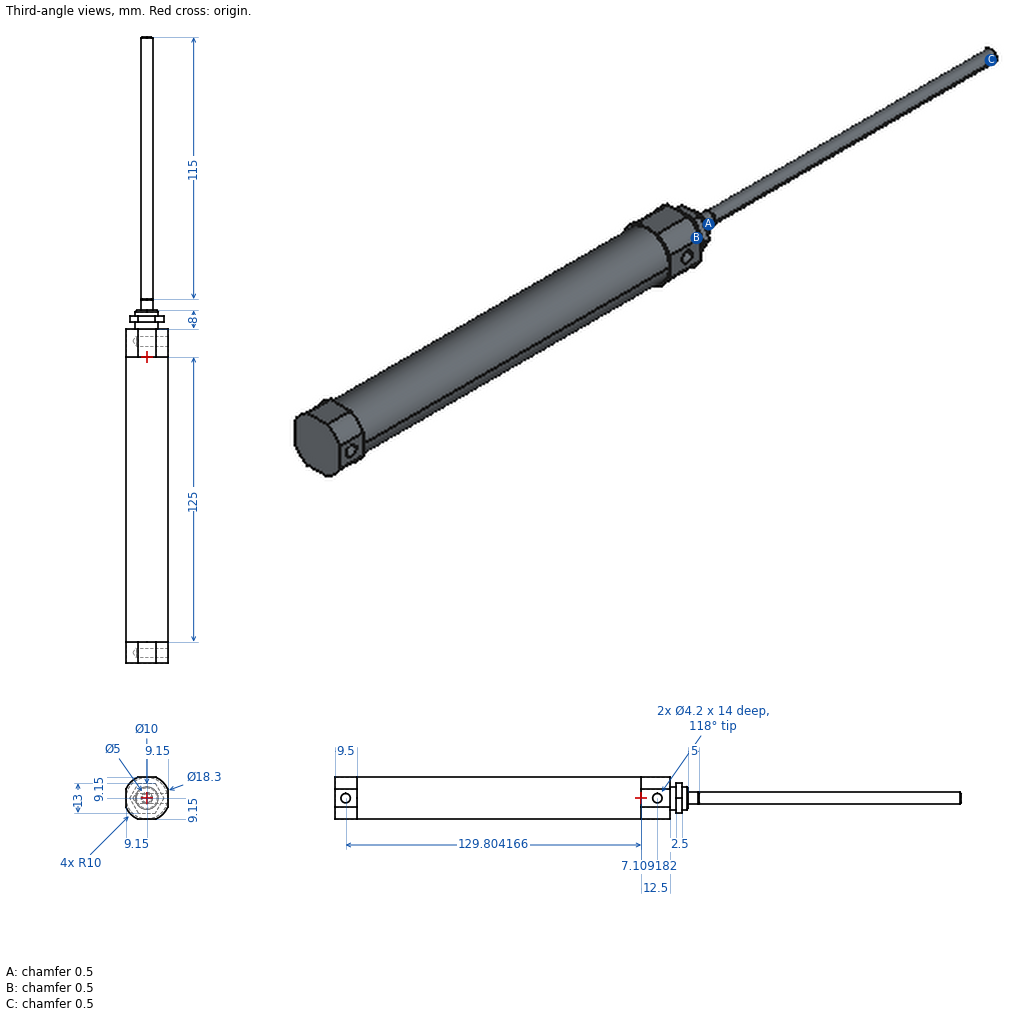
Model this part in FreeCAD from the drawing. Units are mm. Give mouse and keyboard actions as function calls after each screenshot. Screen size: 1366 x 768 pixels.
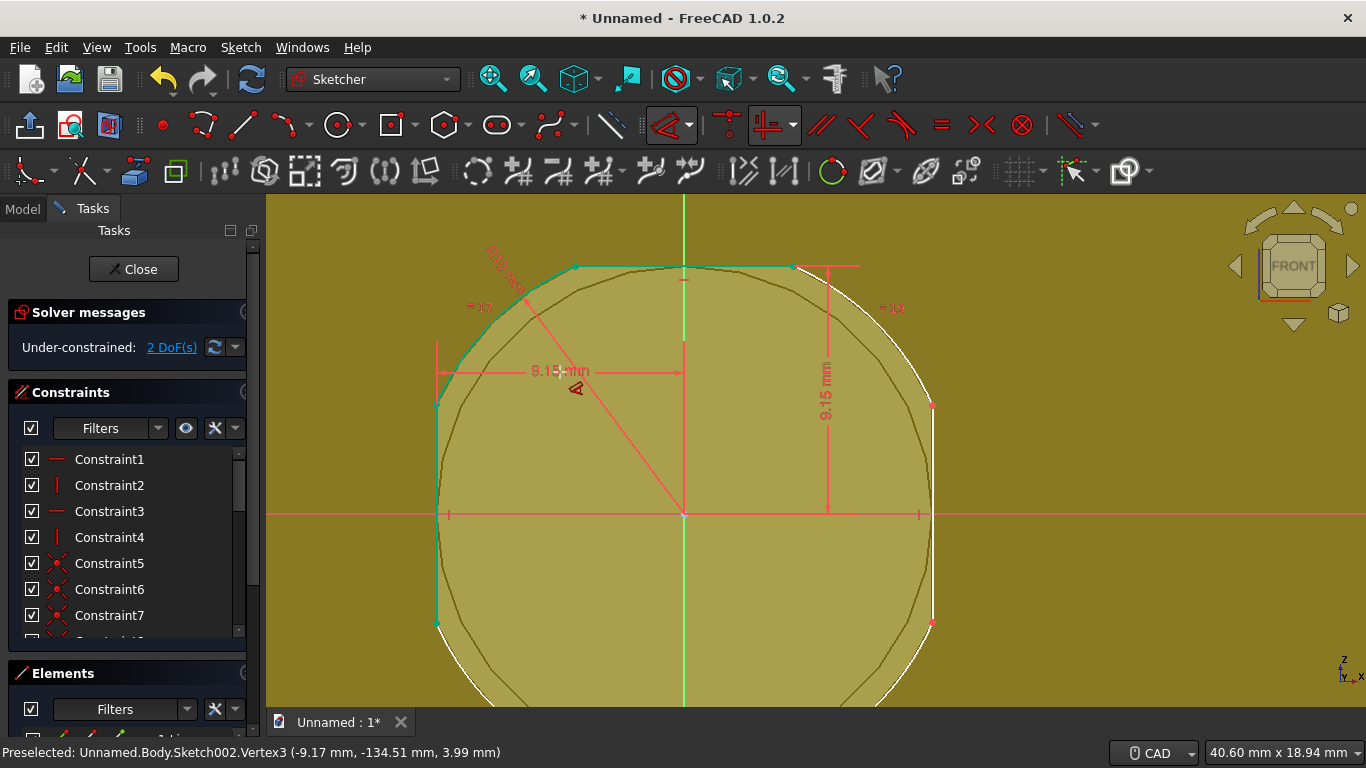
scroll(876, 321, down, 2)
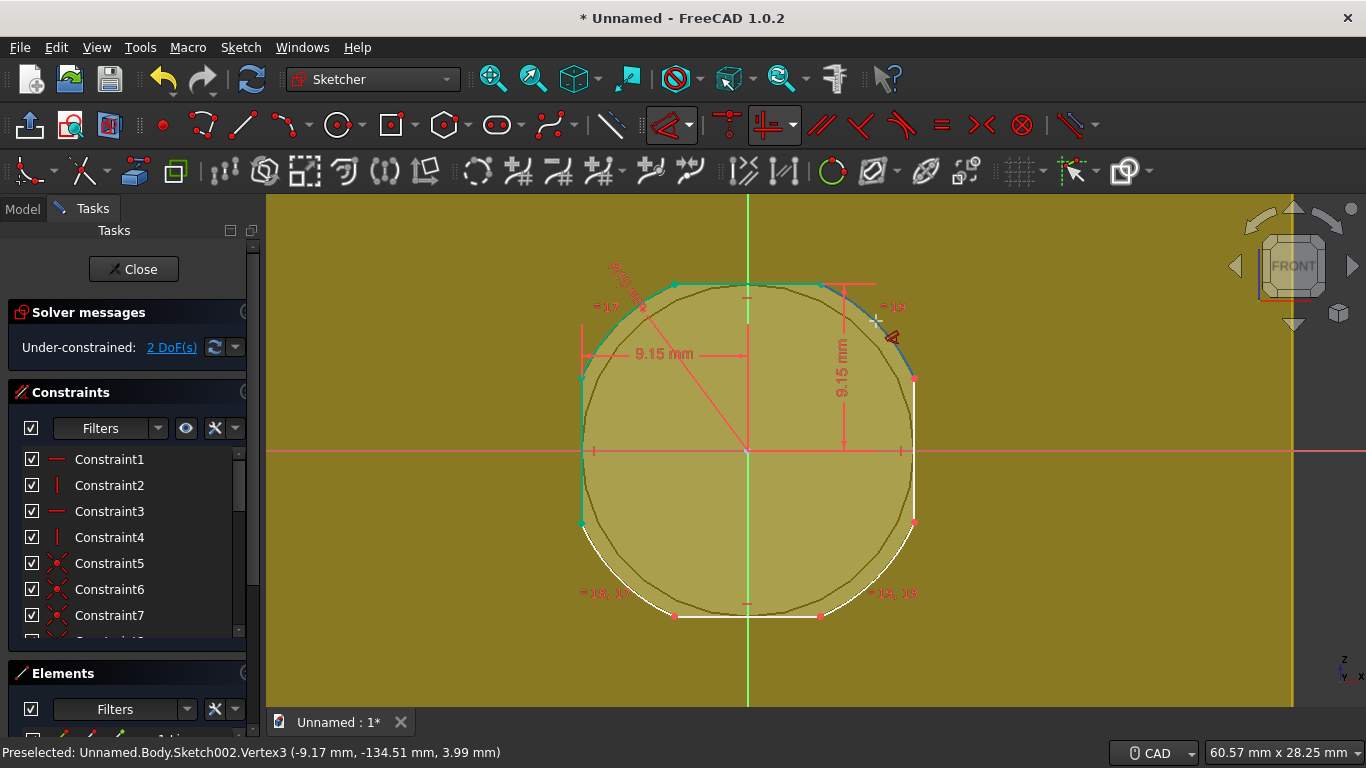
click(675, 617)
click(641, 534)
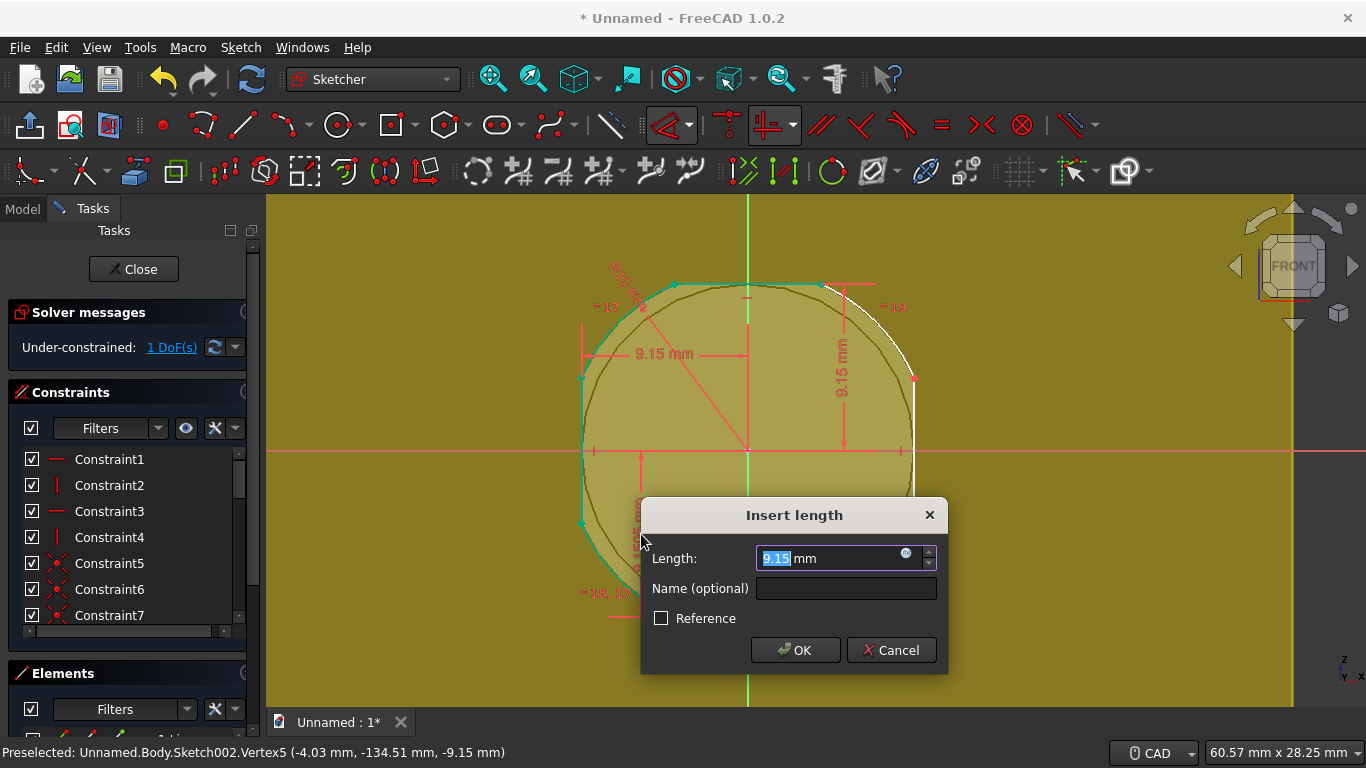
text(9.15)
key(Return)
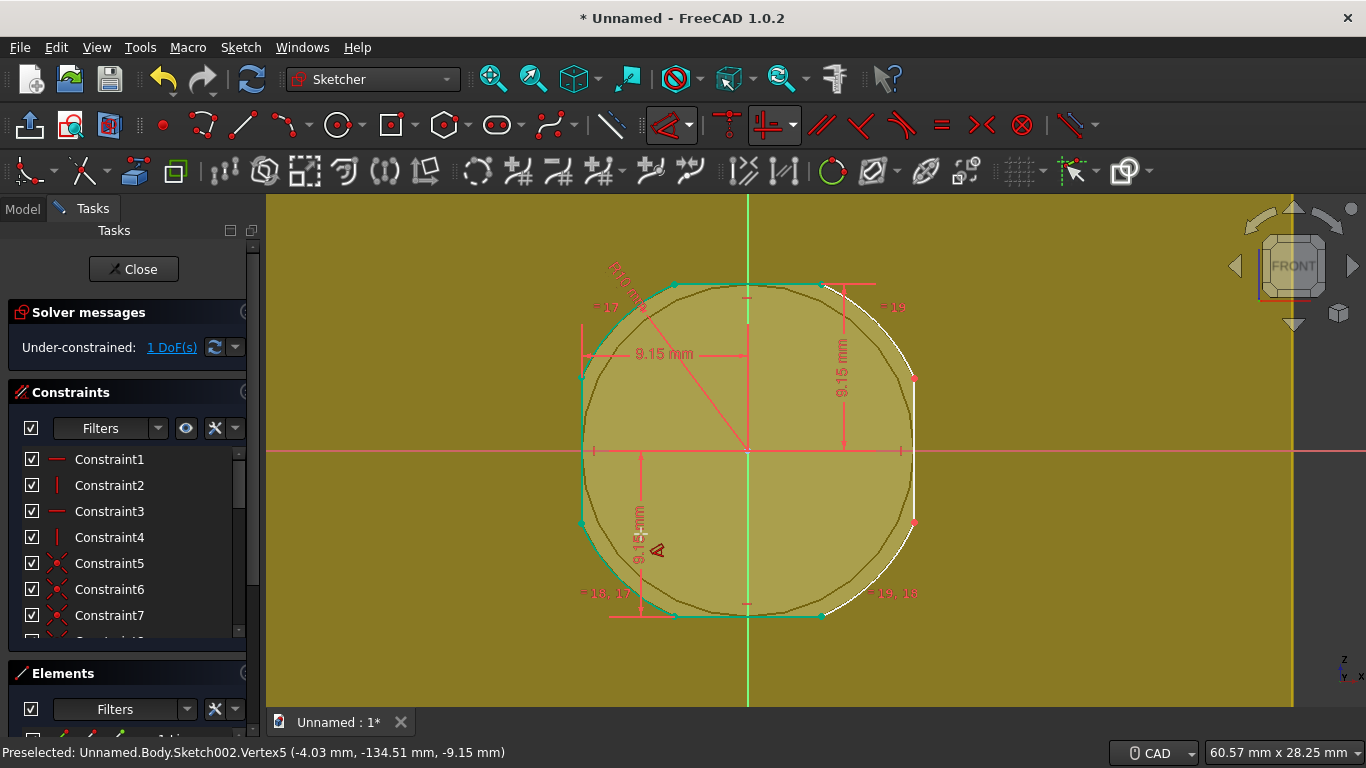
click(914, 523)
click(831, 557)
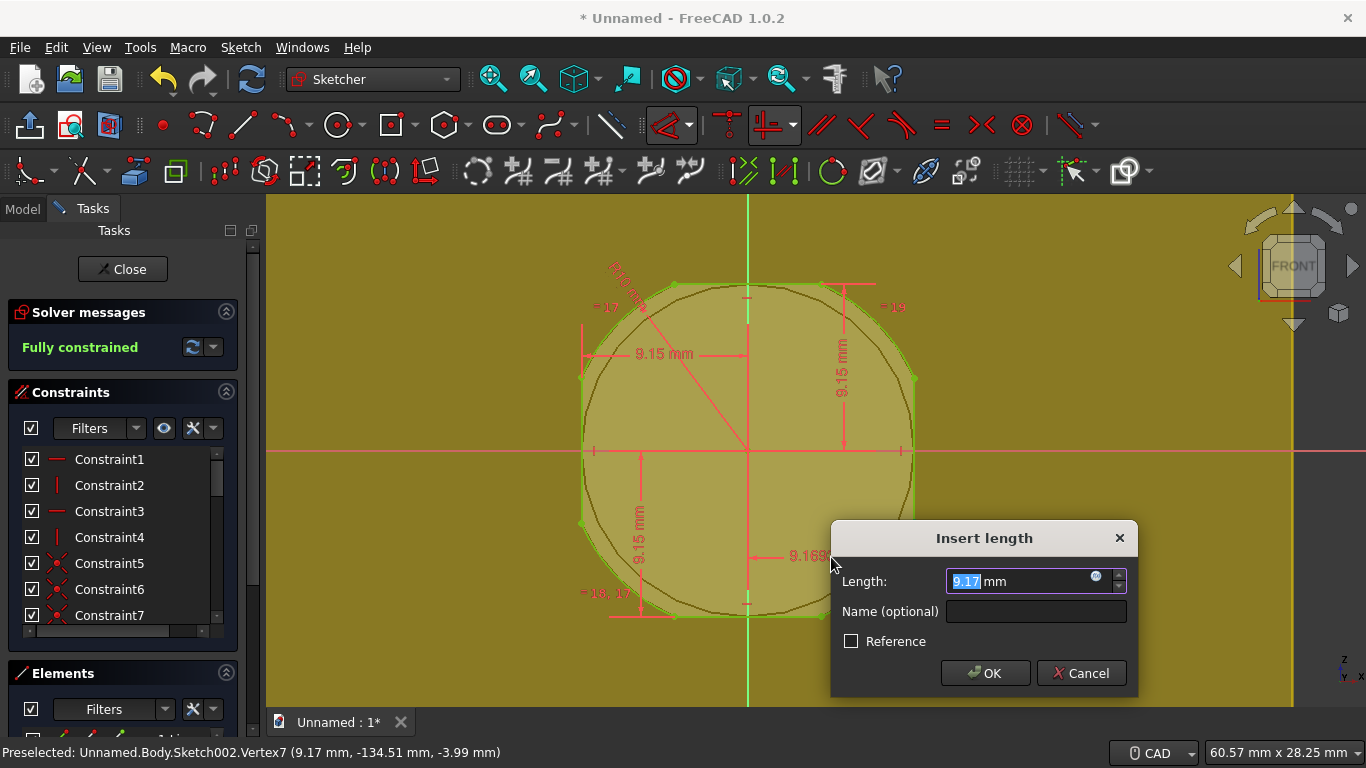
text(9.15)
key(Return)
key(Escape)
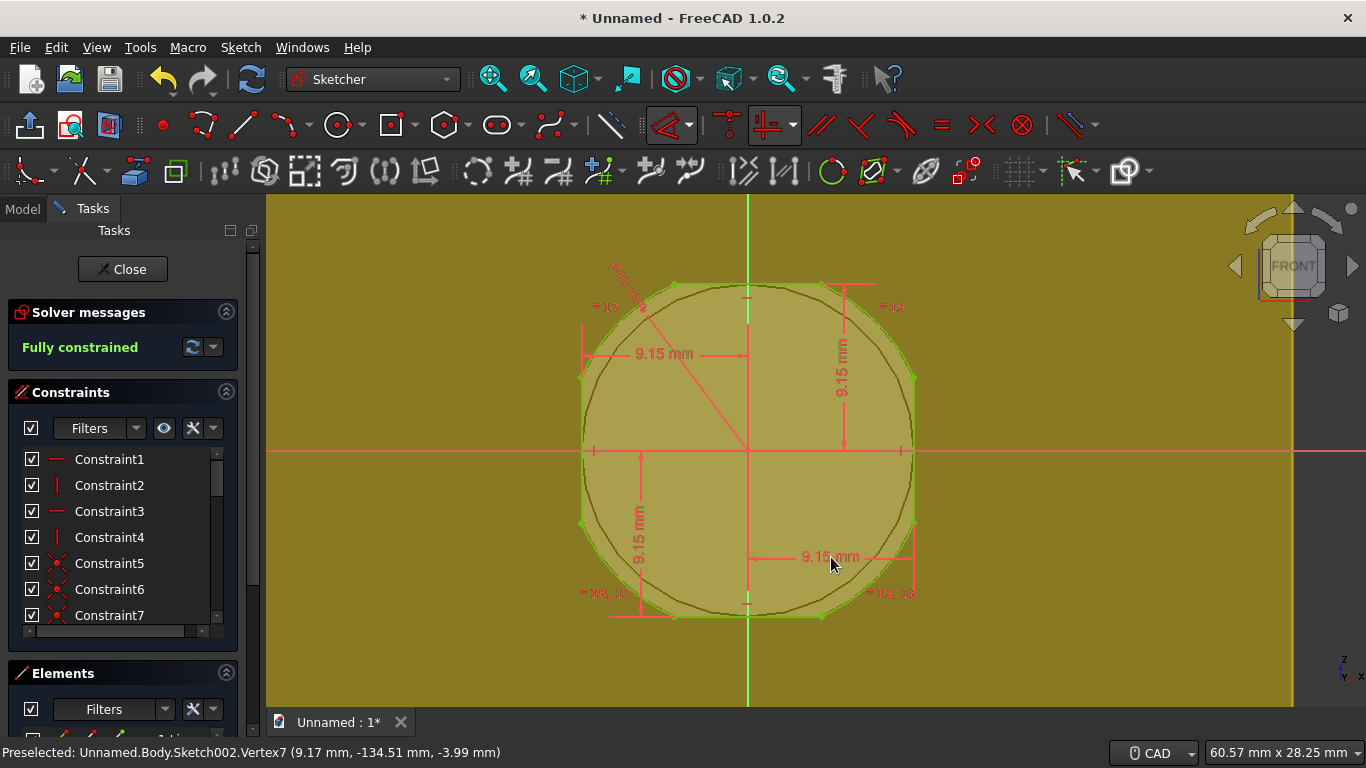
click(123, 269)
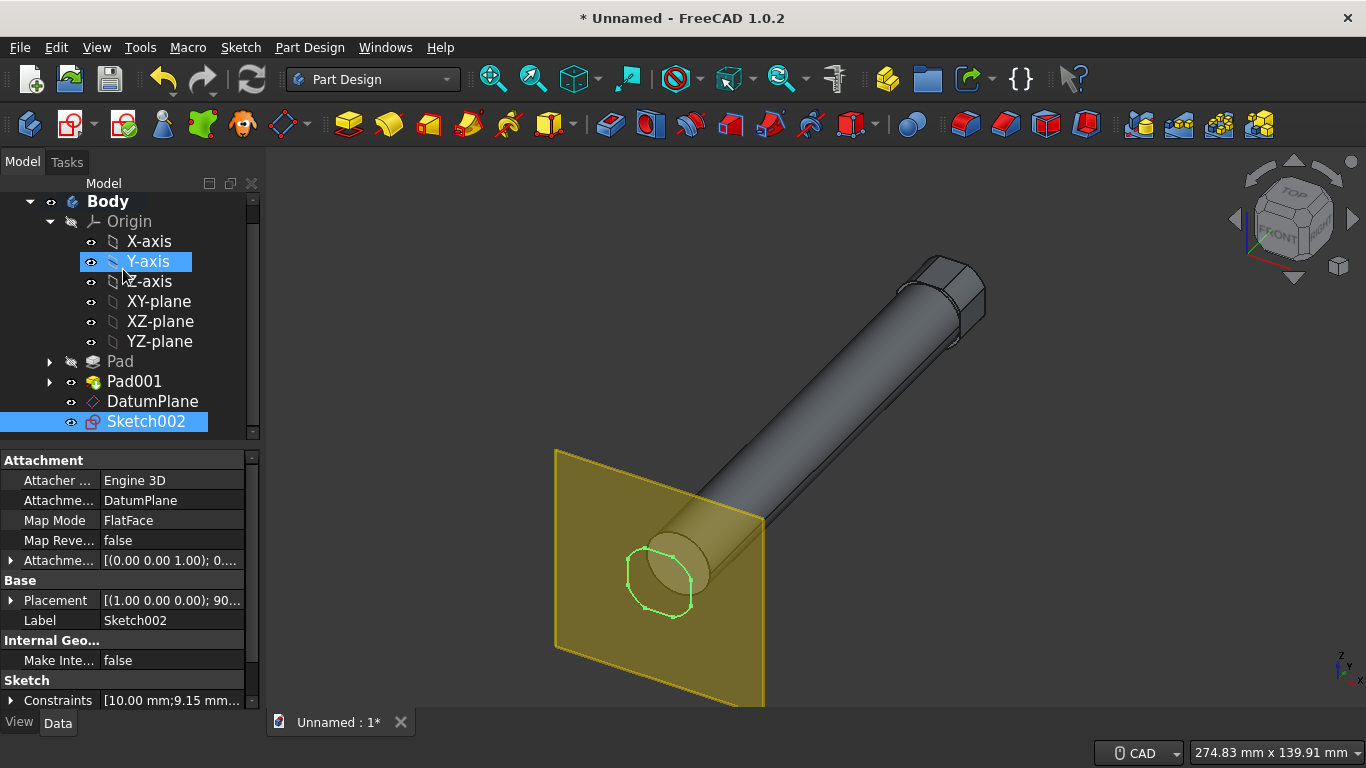
click(350, 124)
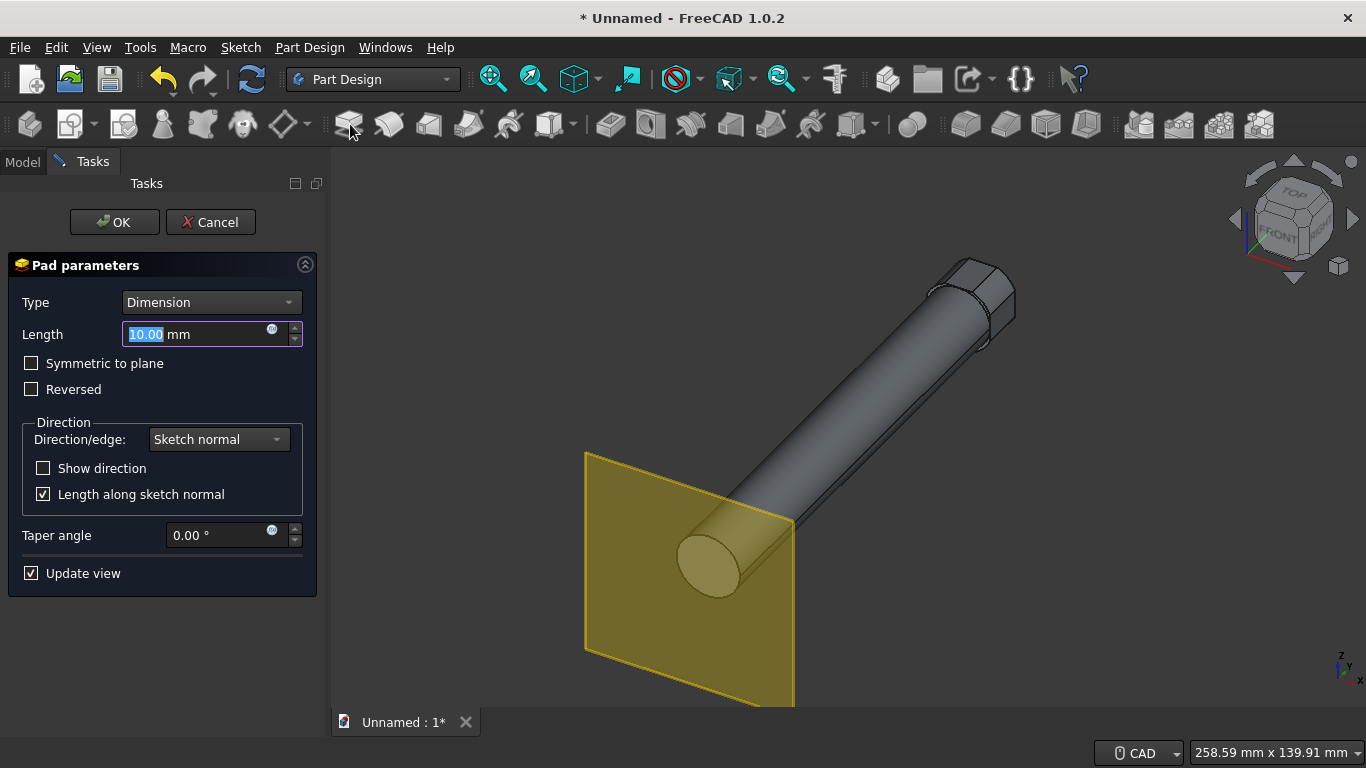
text(9.5)
key(Tab)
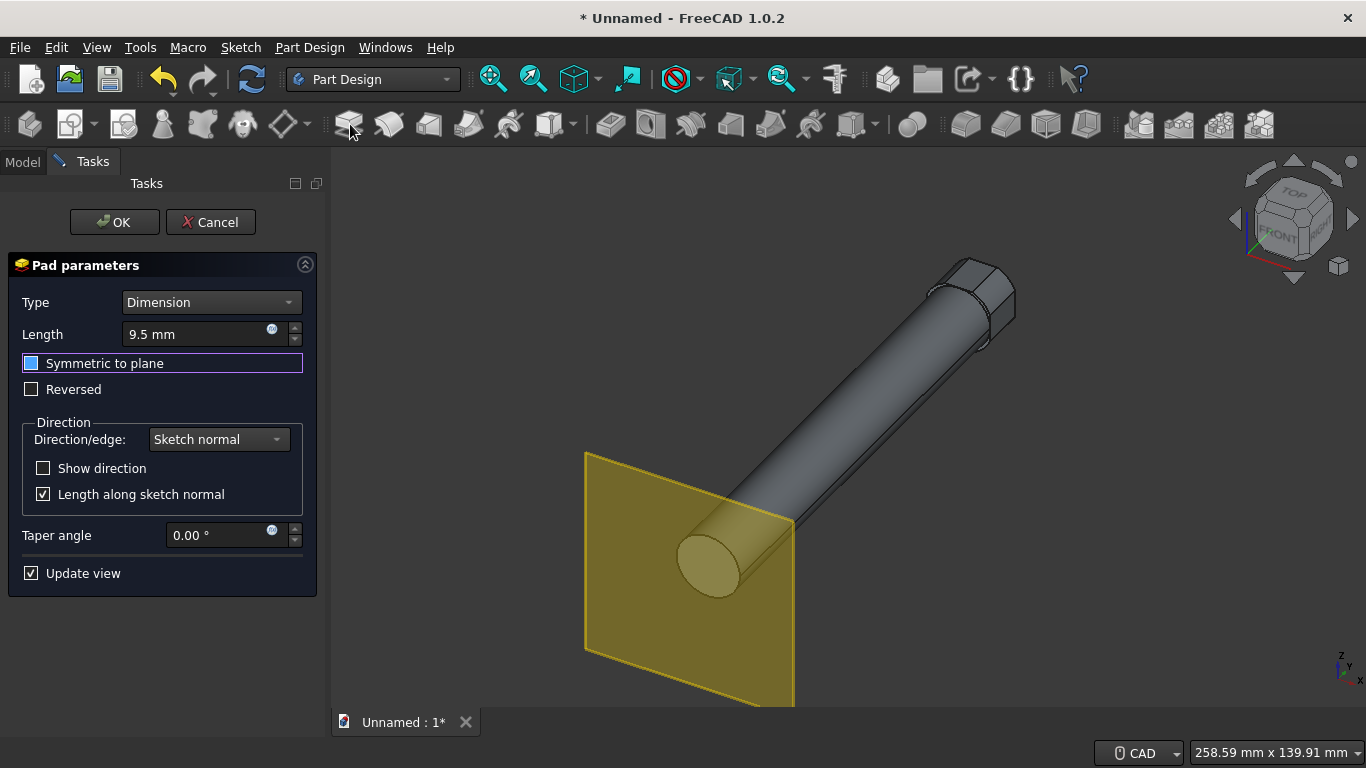
click(30, 389)